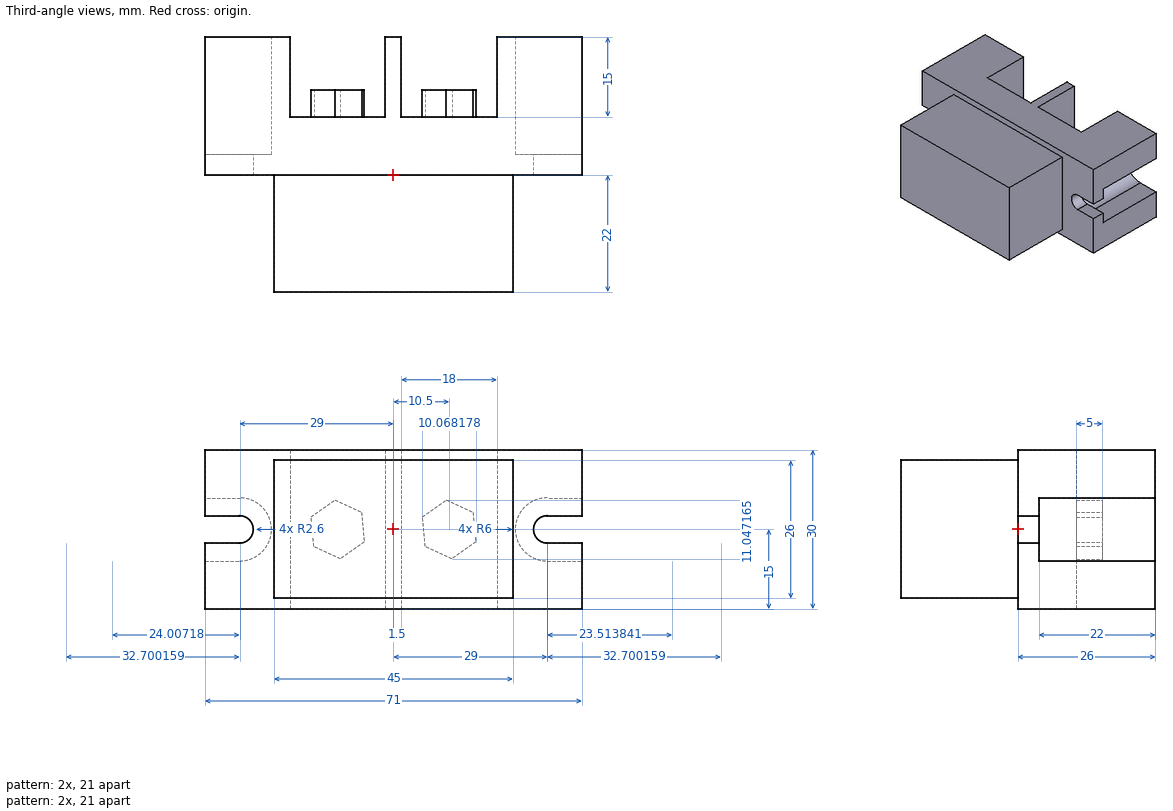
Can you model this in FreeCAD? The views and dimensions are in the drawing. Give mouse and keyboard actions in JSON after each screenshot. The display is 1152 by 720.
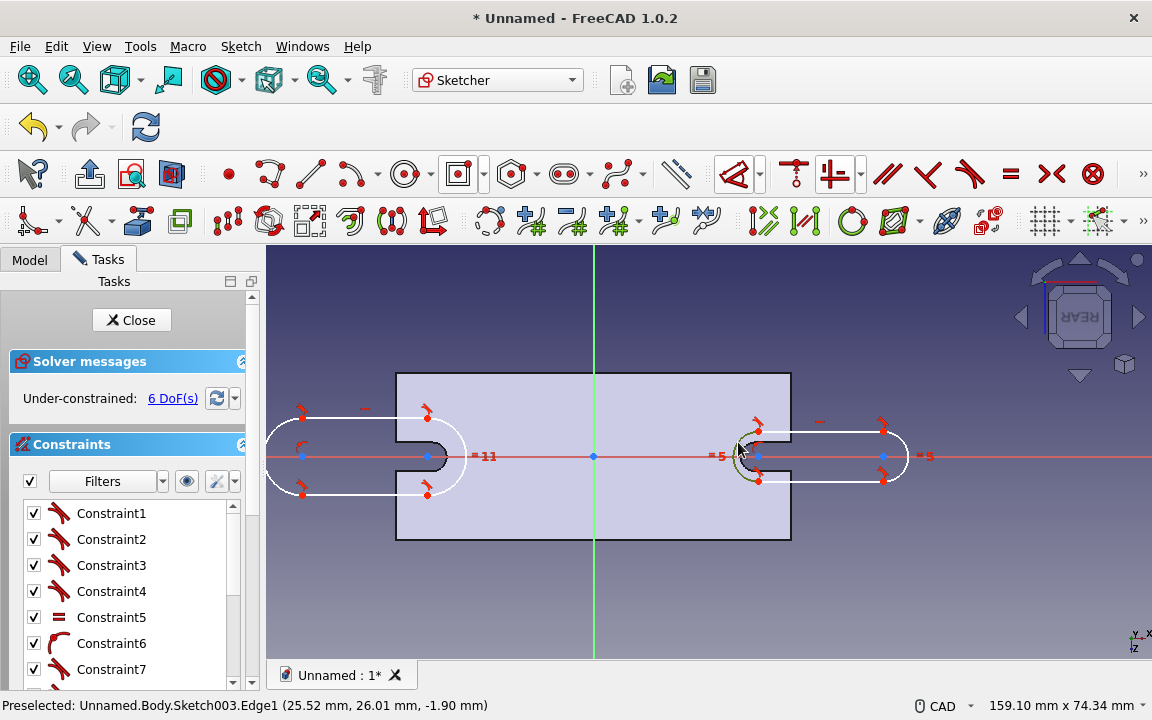
{"action": "scroll", "coordinate": [858, 430], "scroll_direction": "down", "scroll_amount": 1}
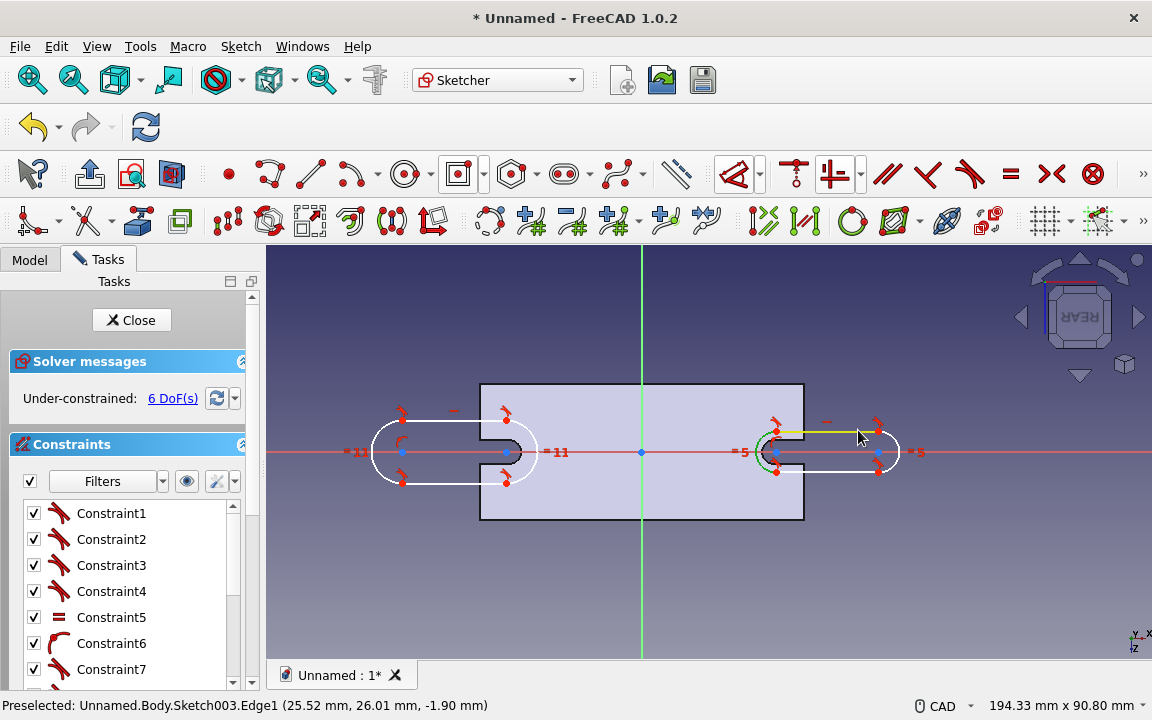
{"action": "left_click", "coordinate": [378, 434]}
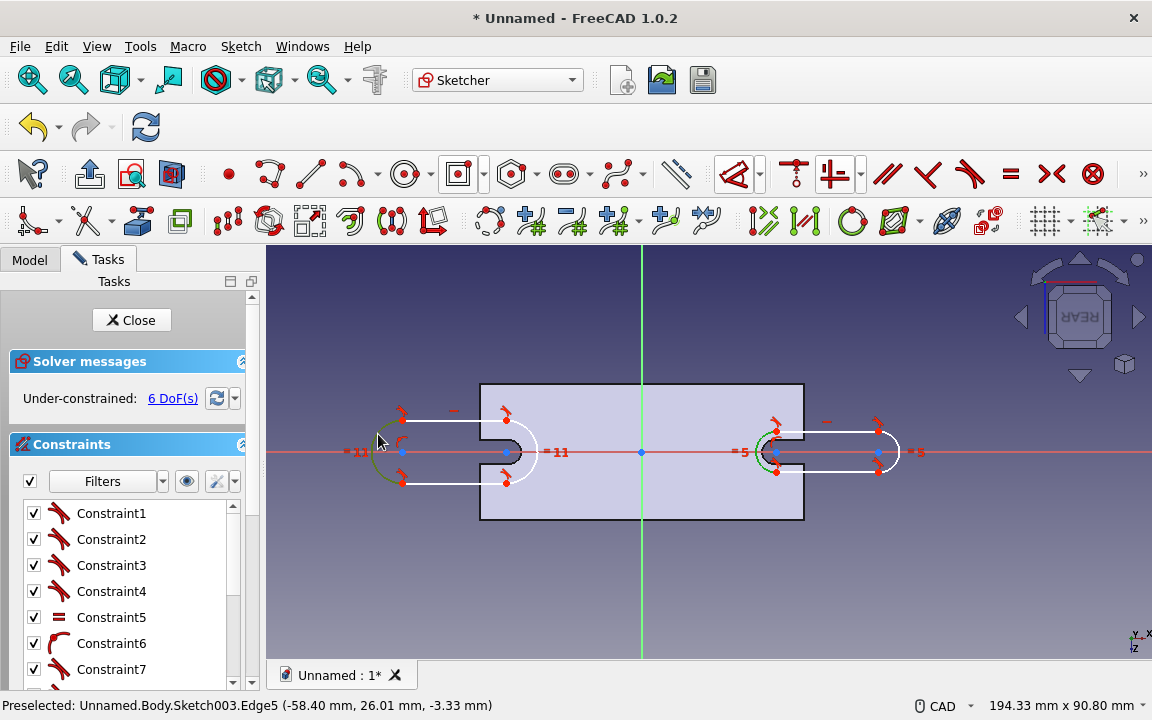
{"action": "left_click", "coordinate": [1011, 174]}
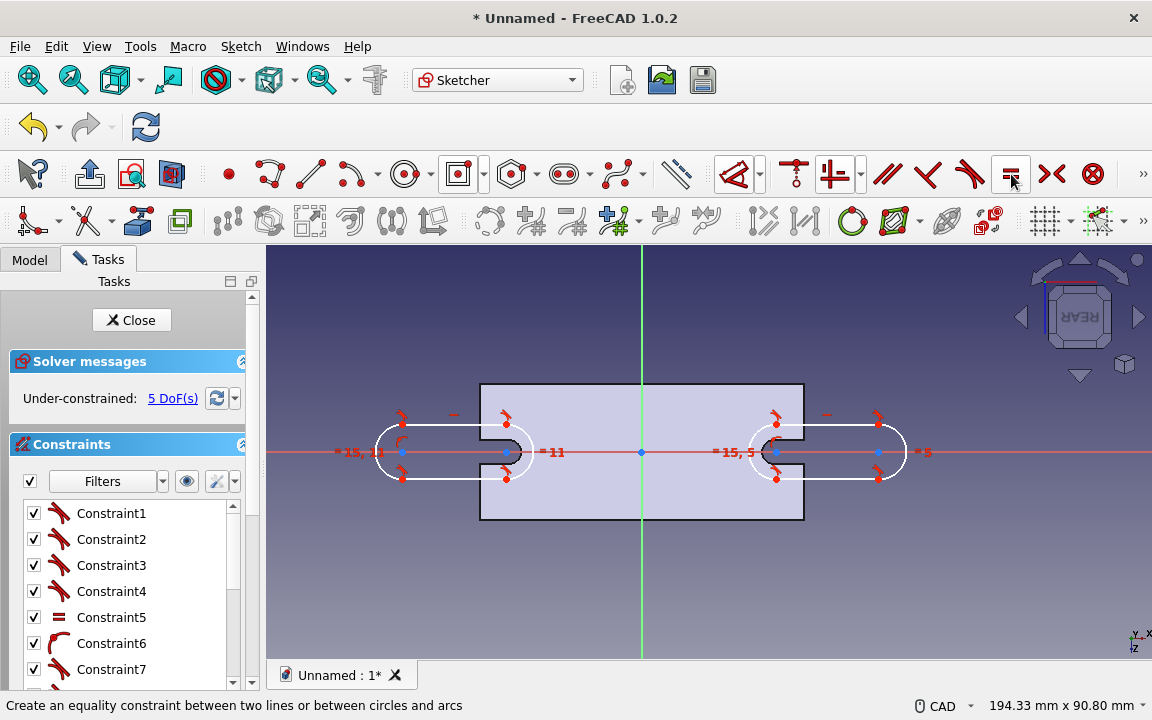
{"action": "scroll", "coordinate": [754, 436], "scroll_direction": "up", "scroll_amount": 2}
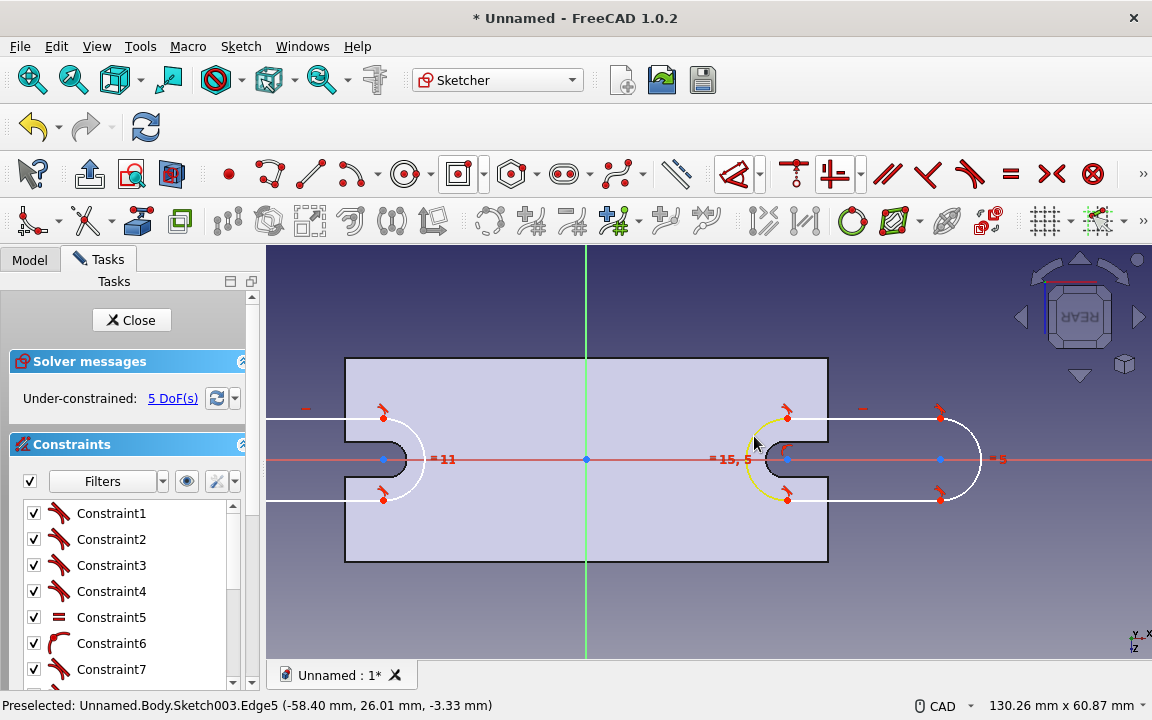
{"action": "left_click", "coordinate": [754, 436]}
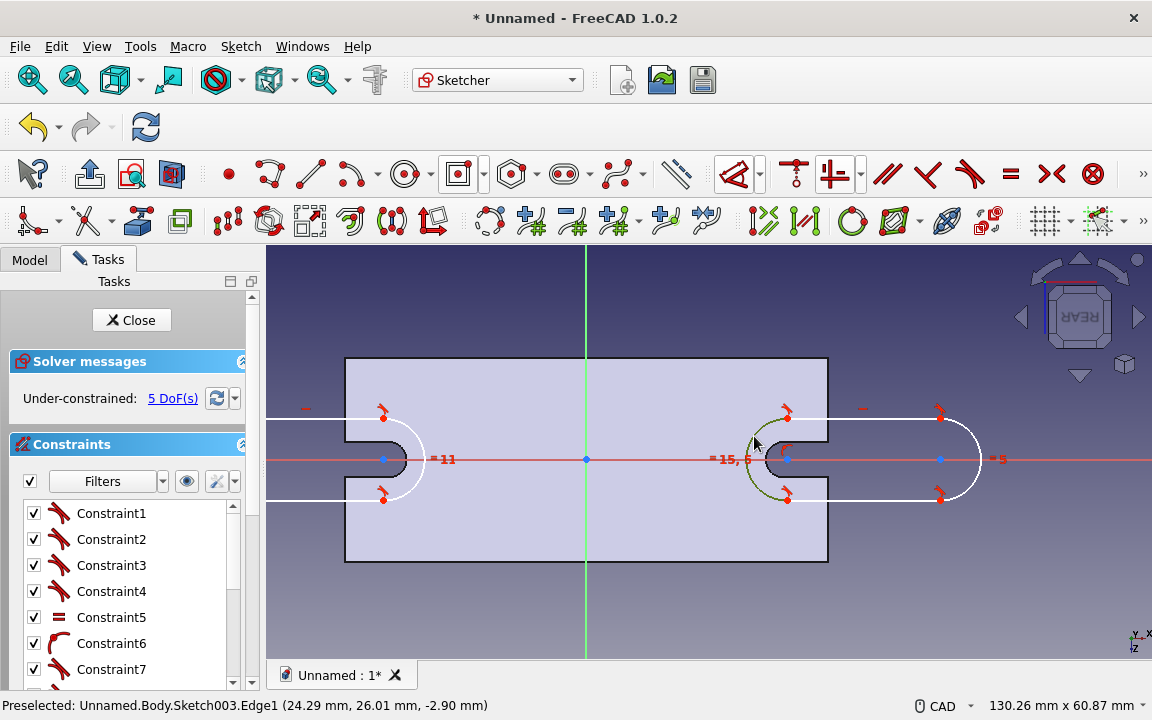
{"action": "key", "text": "k r"}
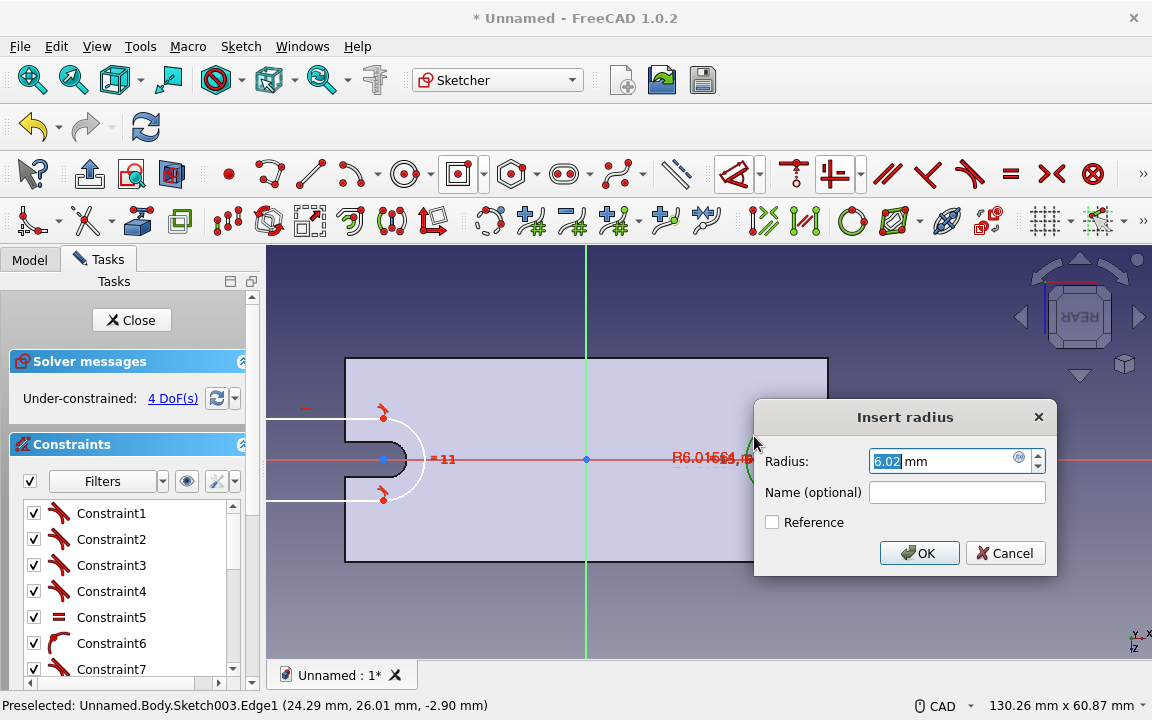
{"action": "type", "text": "6"}
{"action": "key", "text": "Return"}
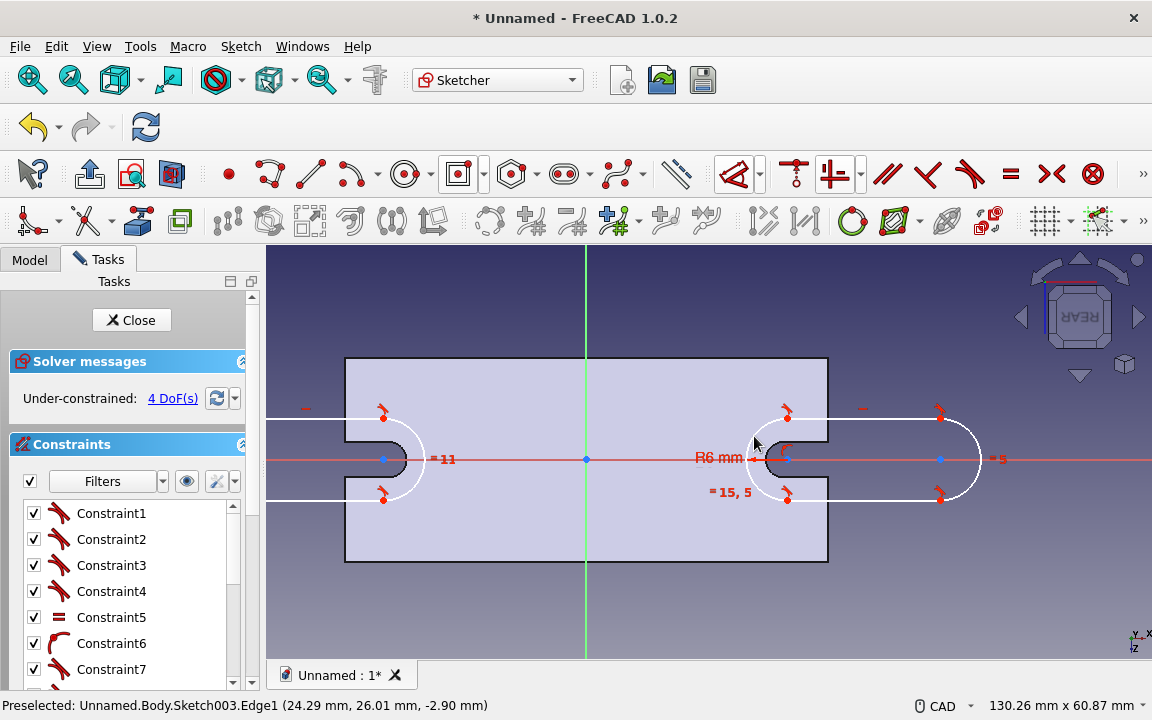
{"action": "left_click", "coordinate": [787, 419]}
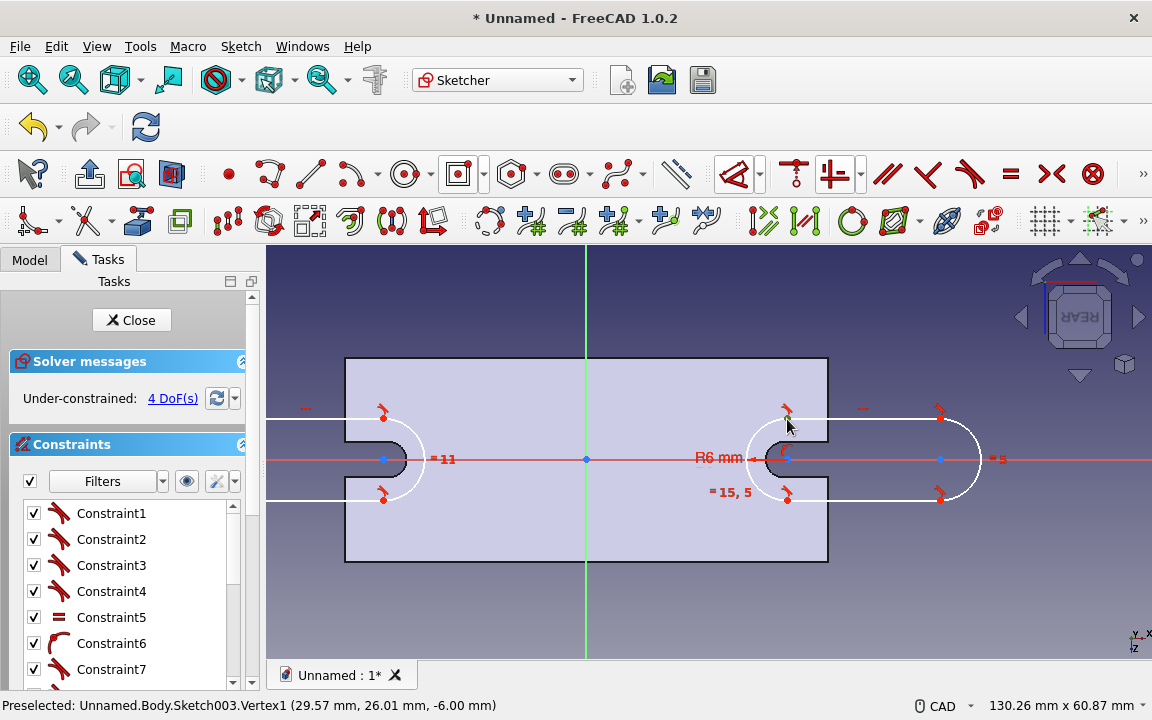
{"action": "key", "text": "l"}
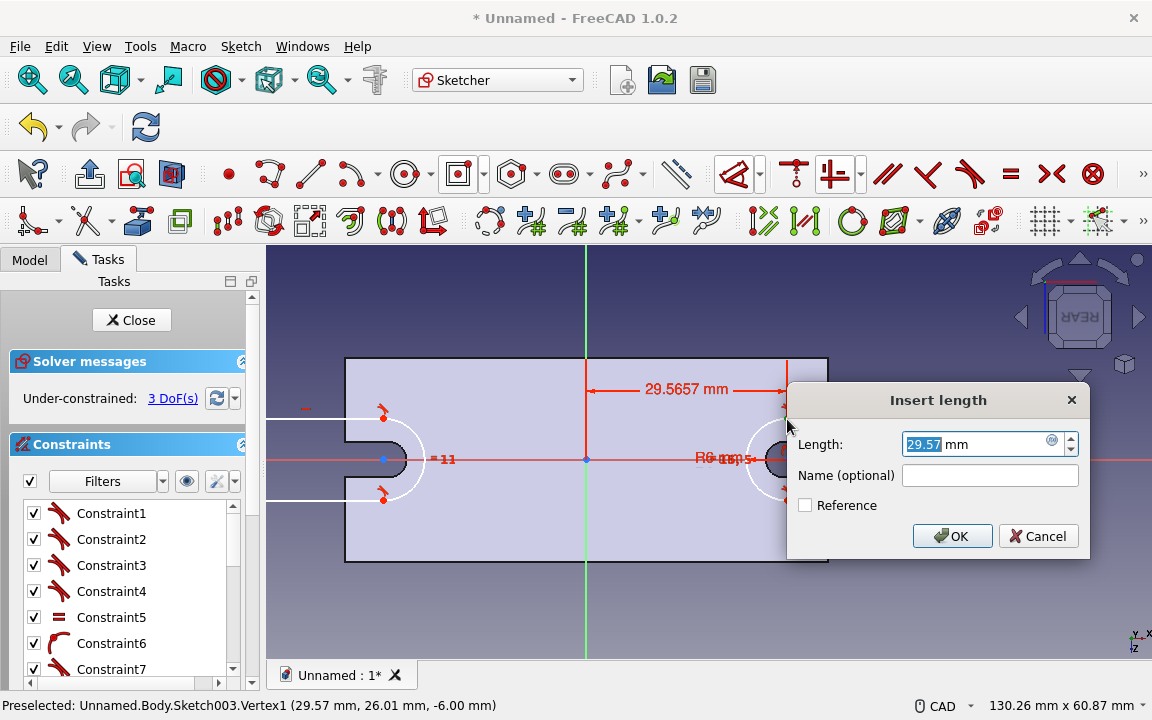
{"action": "type", "text": "29"}
{"action": "key", "text": "Return"}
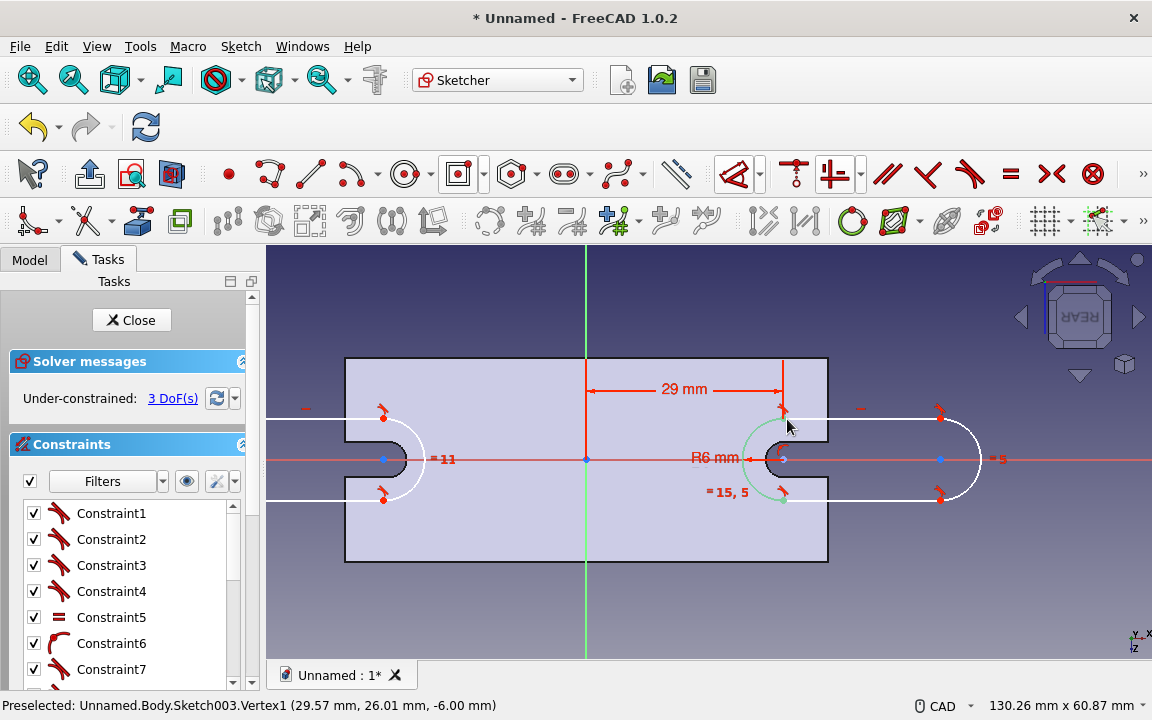
{"action": "left_click", "coordinate": [384, 501]}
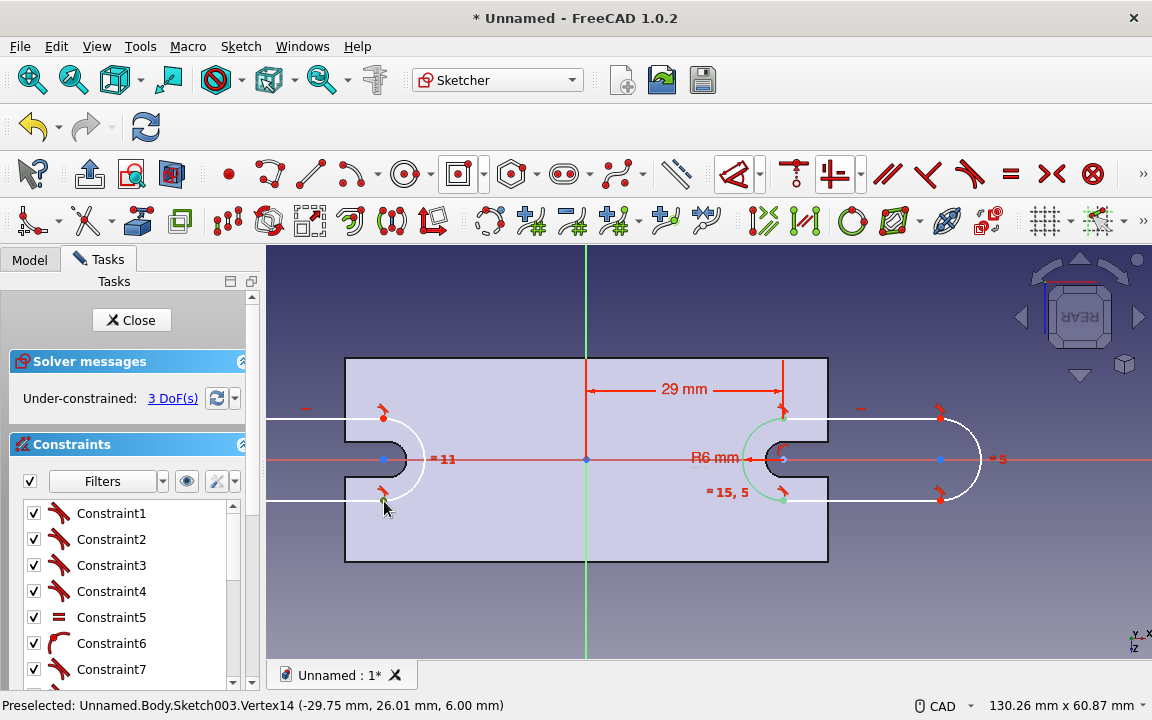
{"action": "left_click", "coordinate": [760, 174]}